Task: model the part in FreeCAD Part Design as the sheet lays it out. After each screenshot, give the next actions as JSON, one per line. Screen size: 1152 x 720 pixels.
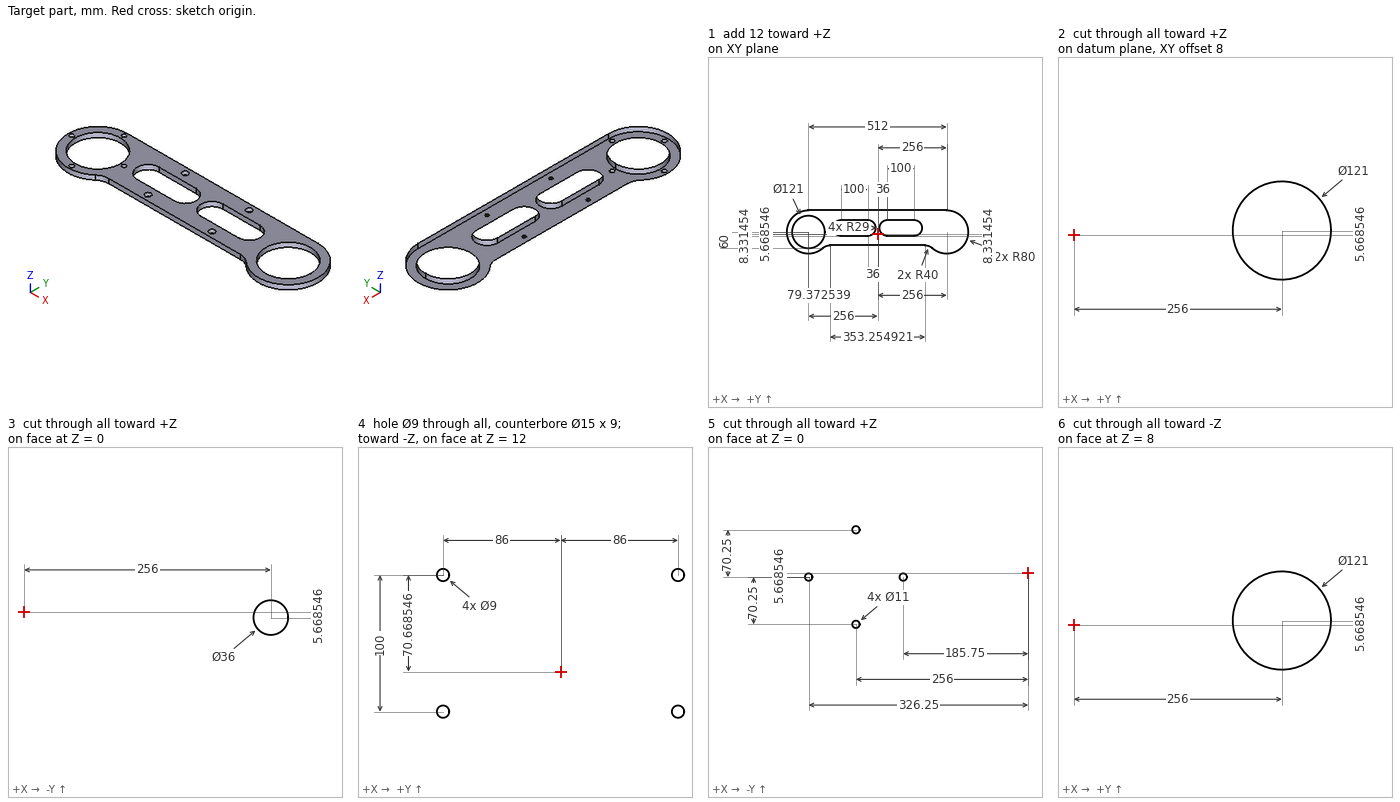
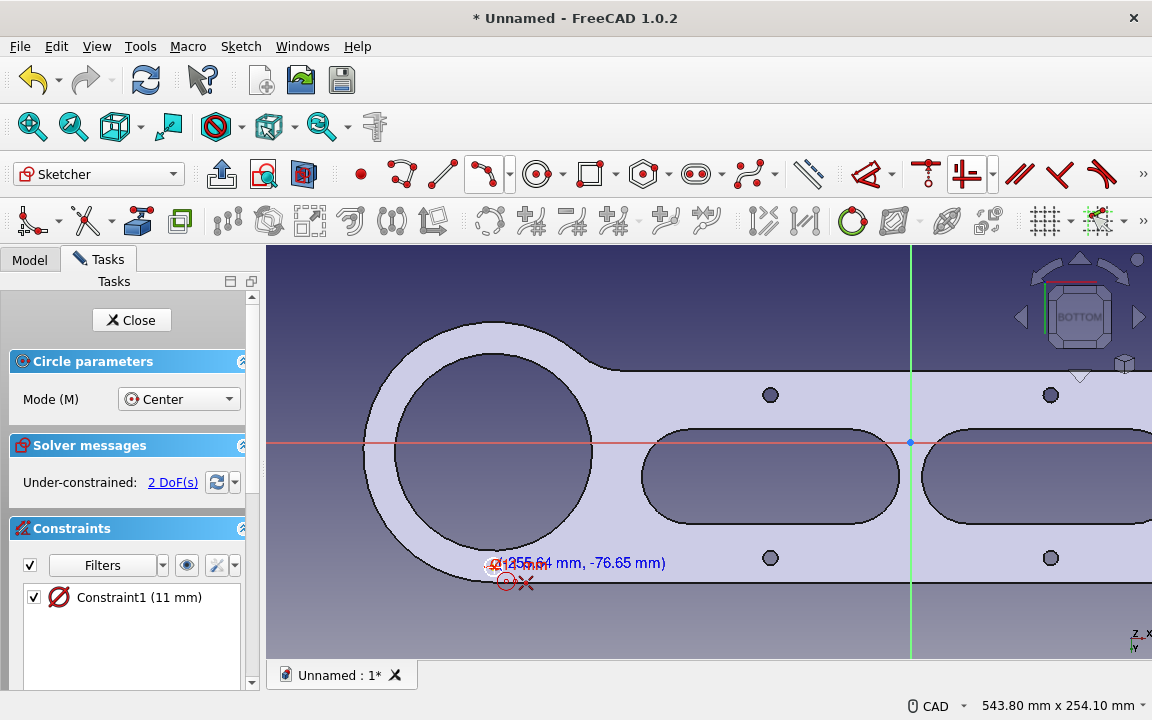
{"action": "scroll", "coordinate": [379, 452], "scroll_direction": "up", "scroll_amount": 5}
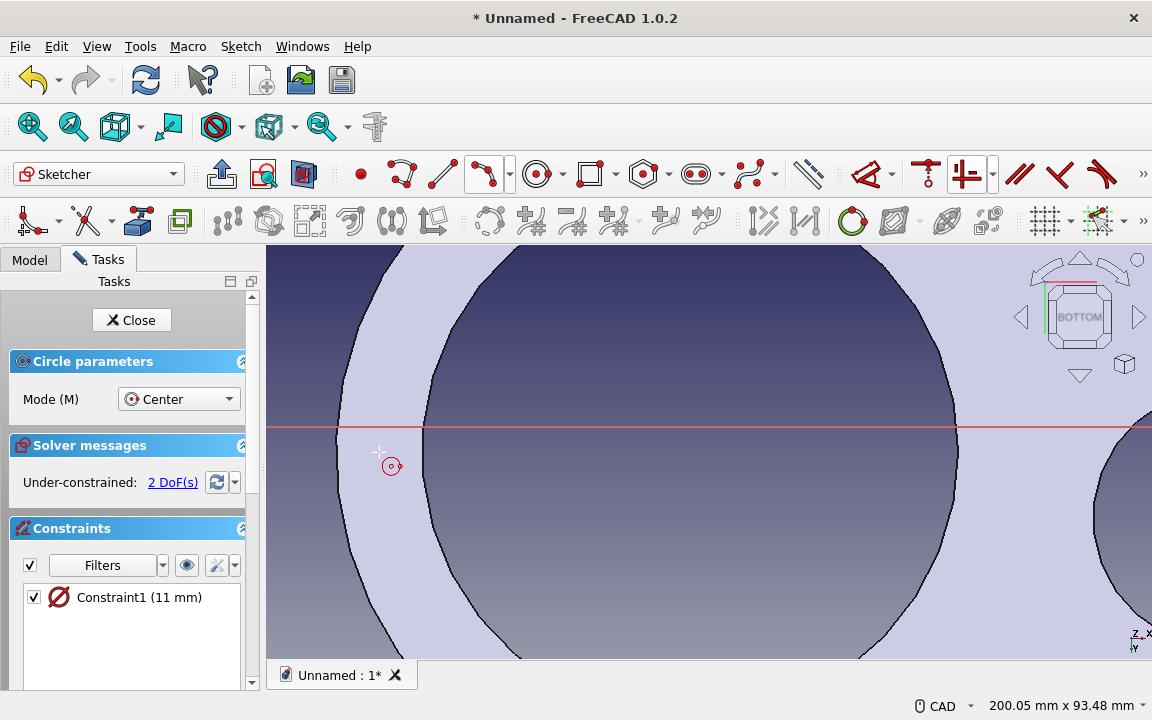
{"action": "left_click", "coordinate": [379, 452]}
{"action": "mouse_move", "coordinate": [396, 469]}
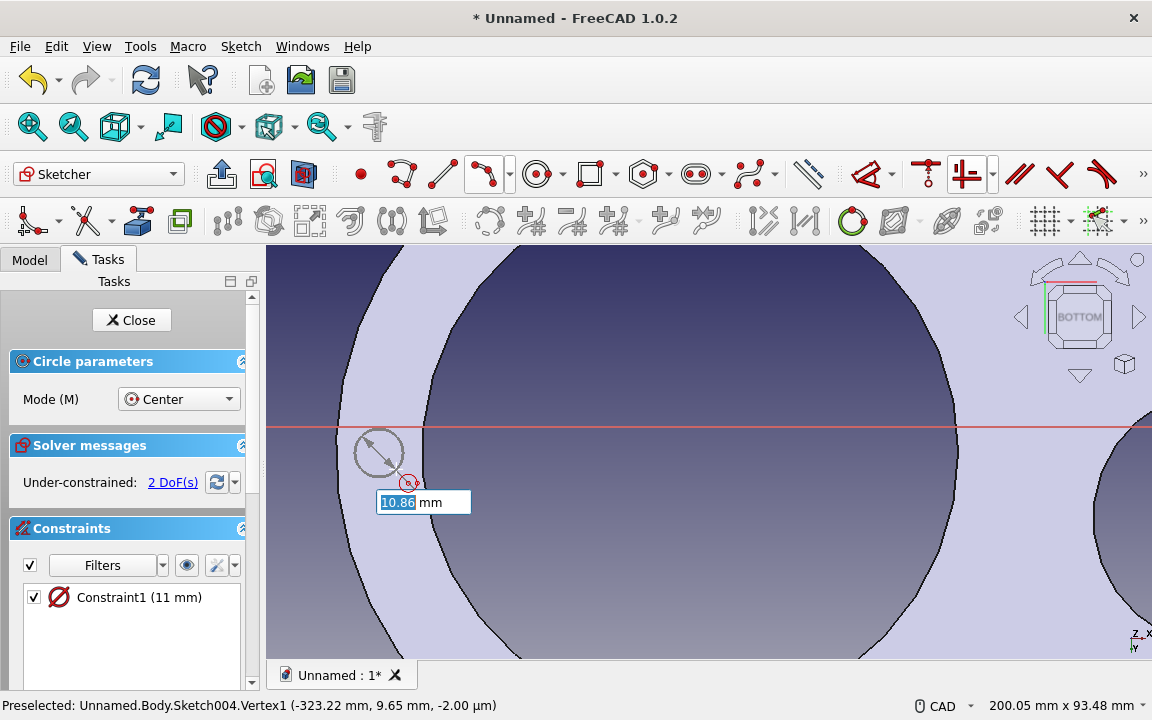
{"action": "type", "text": "11"}
{"action": "key", "text": "Return"}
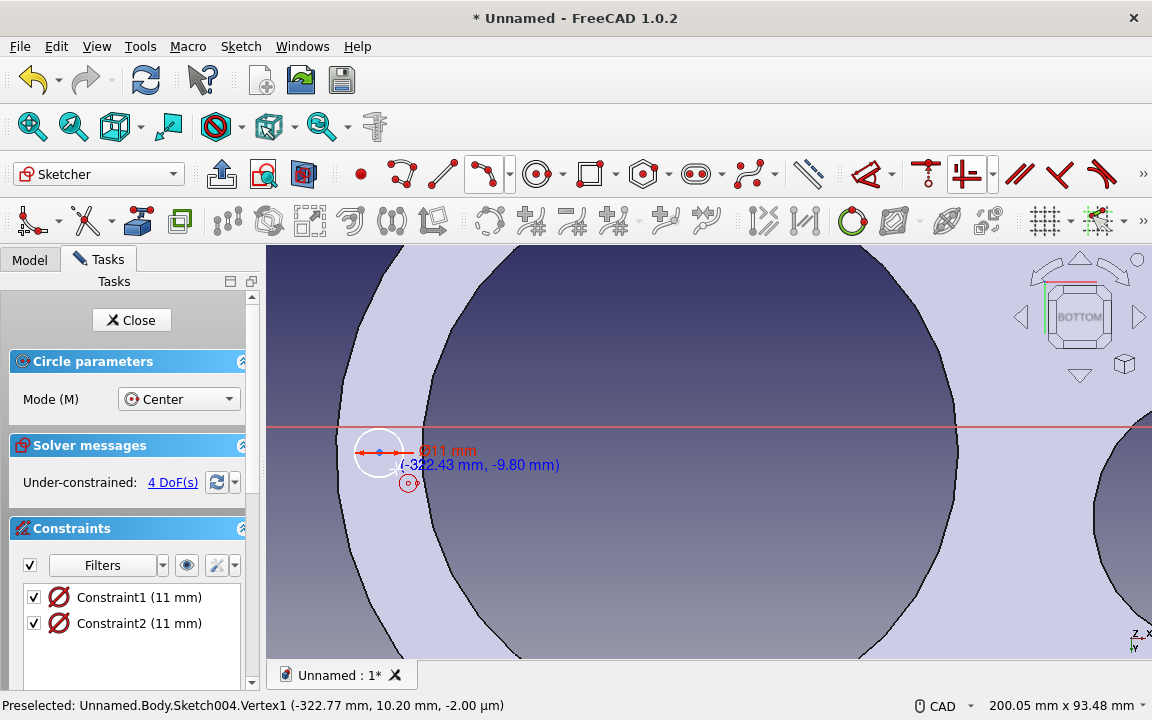
{"action": "scroll", "coordinate": [379, 452], "scroll_direction": "down", "scroll_amount": 5}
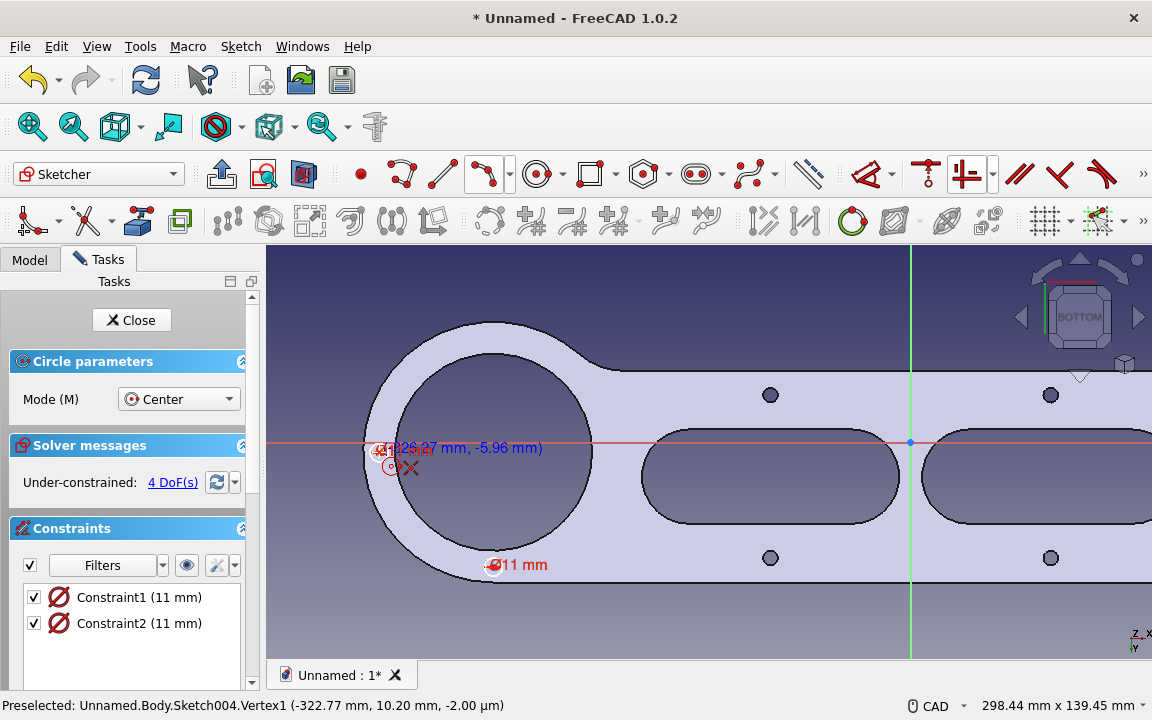
{"action": "scroll", "coordinate": [494, 338], "scroll_direction": "up", "scroll_amount": 5}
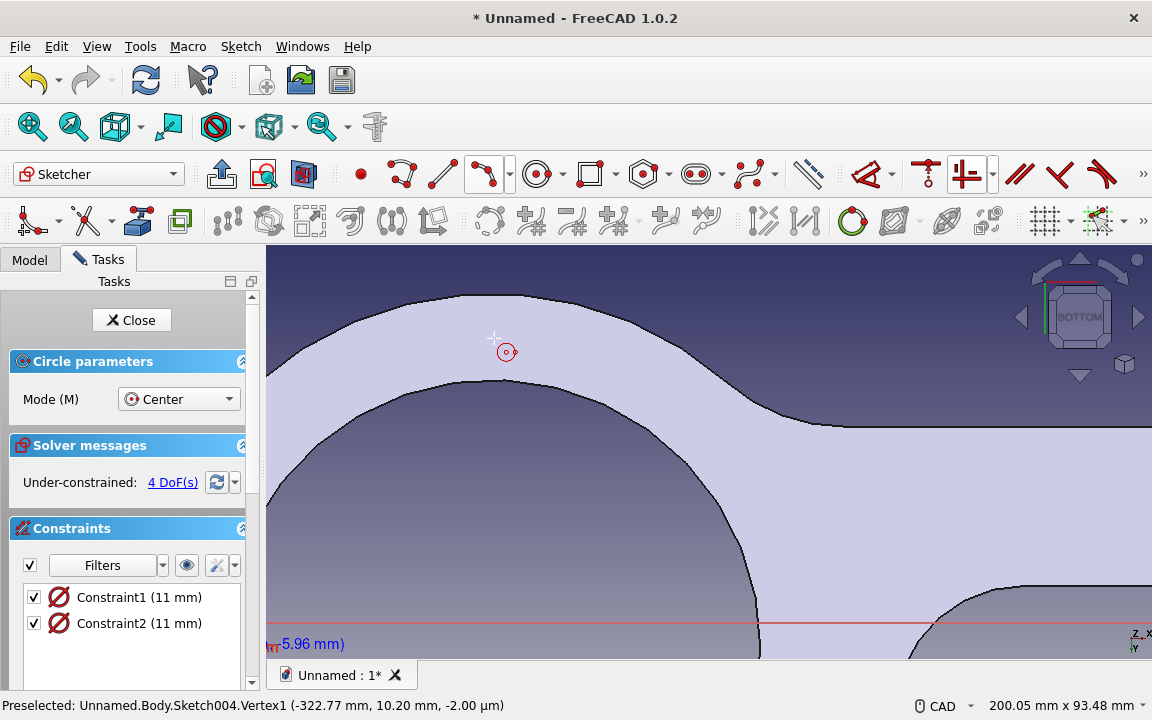
{"action": "left_click", "coordinate": [492, 337]}
{"action": "mouse_move", "coordinate": [510, 320]}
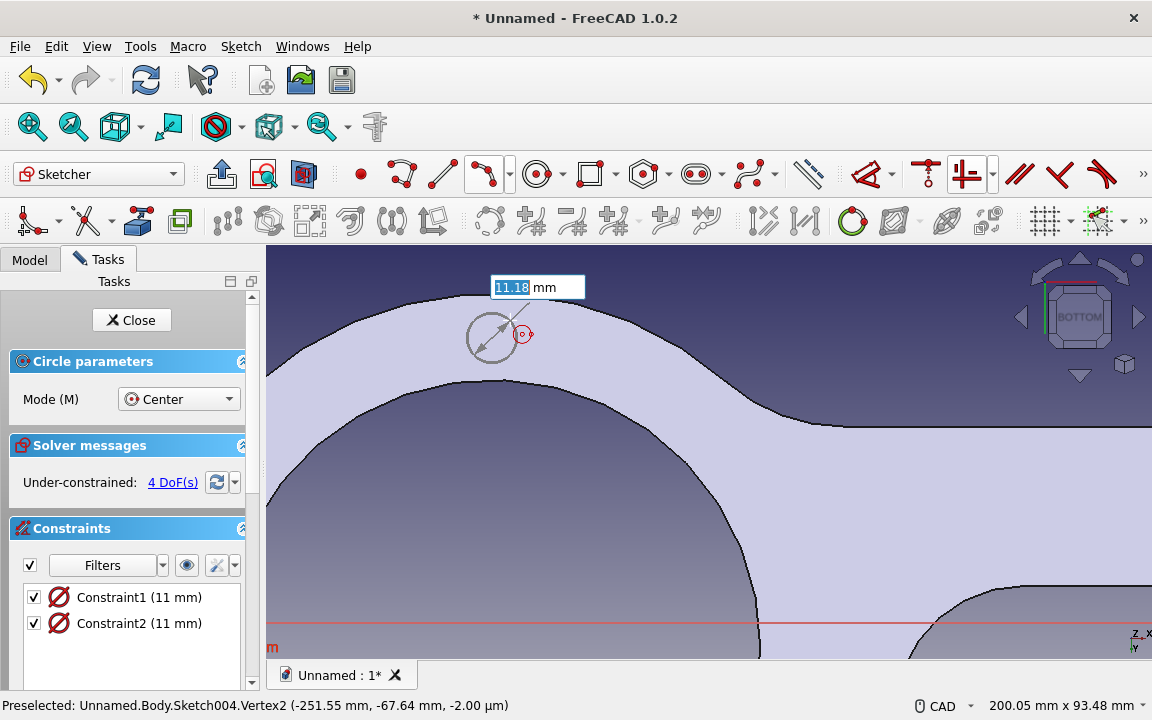
{"action": "type", "text": "11"}
{"action": "key", "text": "Return"}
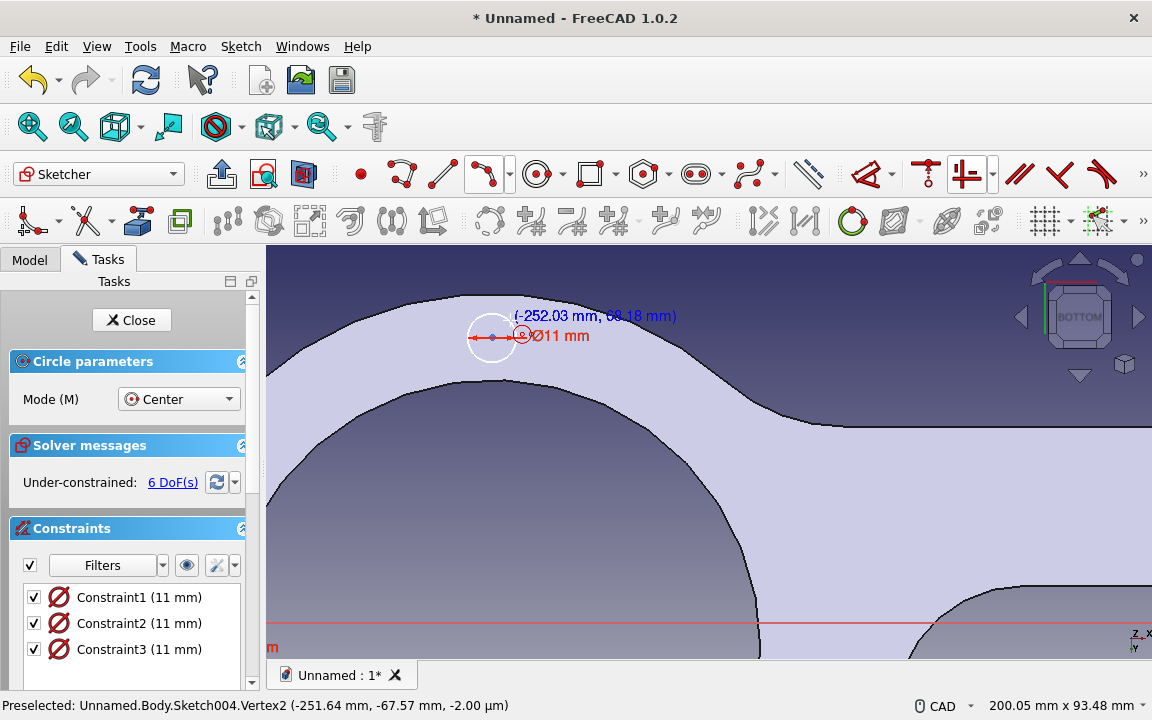
{"action": "scroll", "coordinate": [494, 338], "scroll_direction": "down", "scroll_amount": 5}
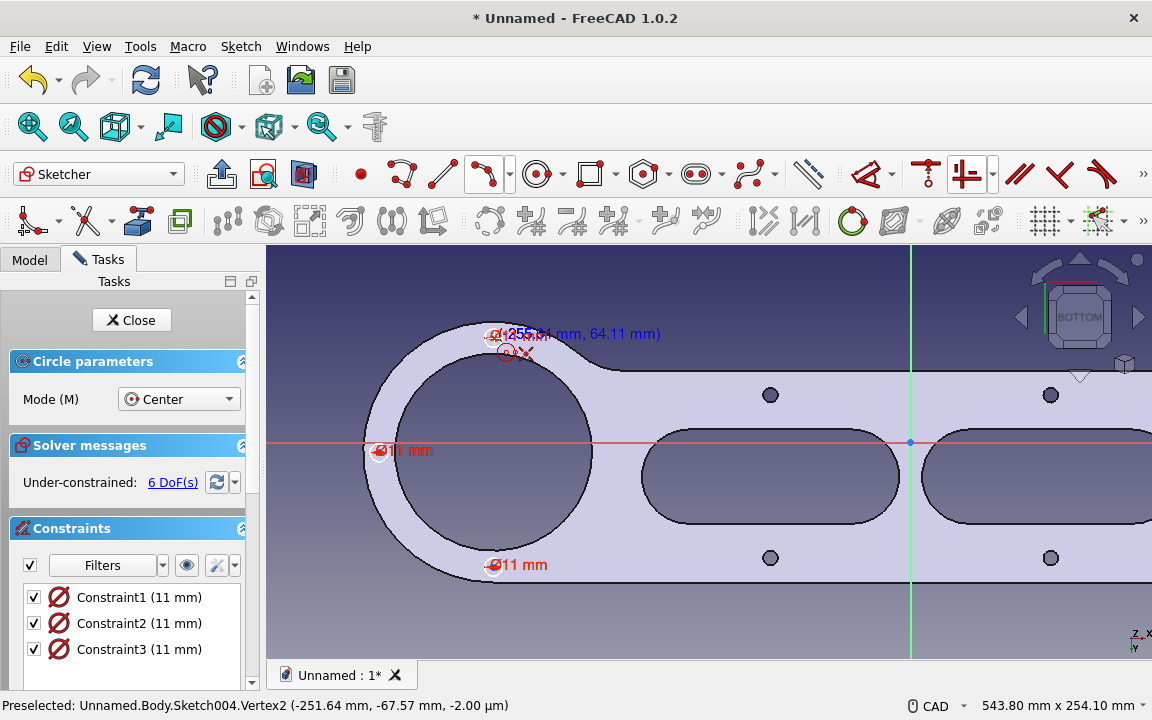
{"action": "scroll", "coordinate": [608, 452], "scroll_direction": "up", "scroll_amount": 5}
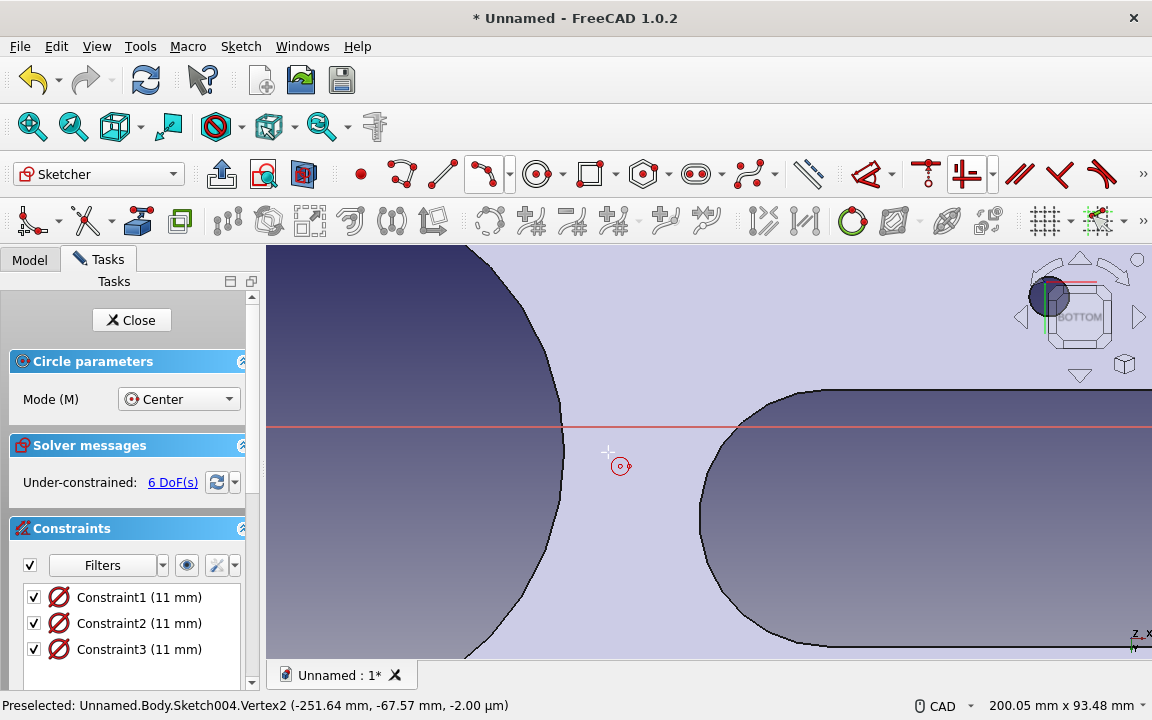
{"action": "left_click", "coordinate": [607, 452]}
{"action": "mouse_move", "coordinate": [625, 469]}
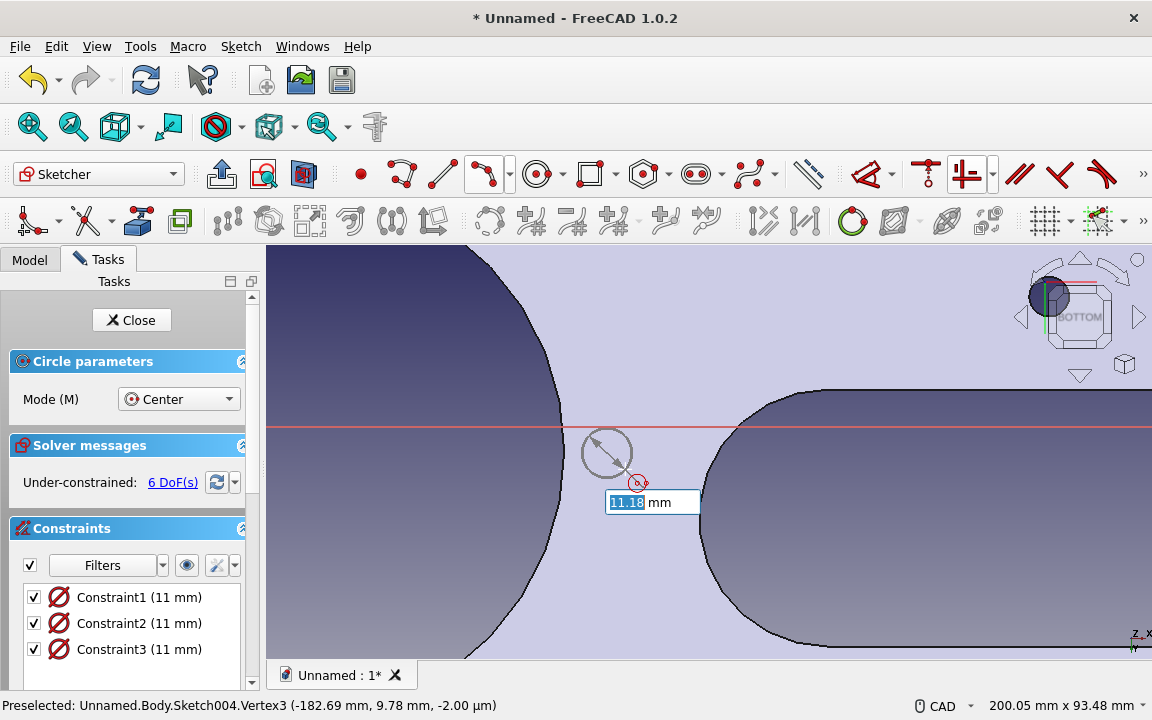
{"action": "type", "text": "11"}
{"action": "key", "text": "Return"}
{"action": "key", "text": "Escape"}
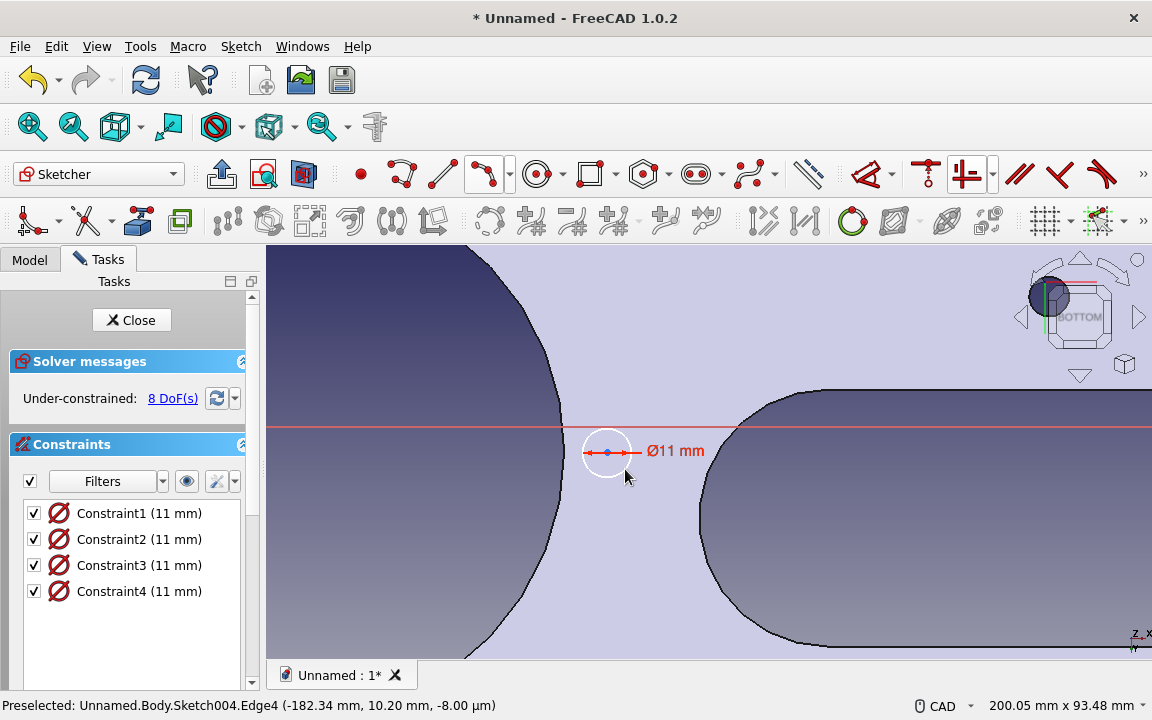
{"action": "scroll", "coordinate": [609, 452], "scroll_direction": "down", "scroll_amount": 5}